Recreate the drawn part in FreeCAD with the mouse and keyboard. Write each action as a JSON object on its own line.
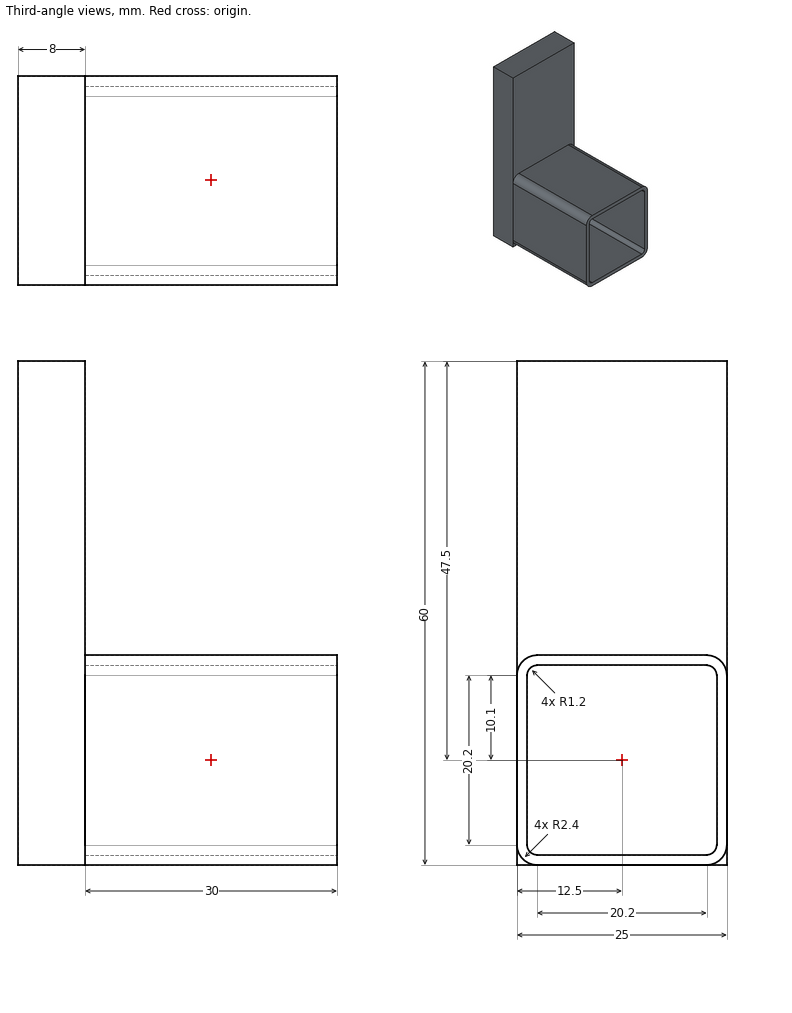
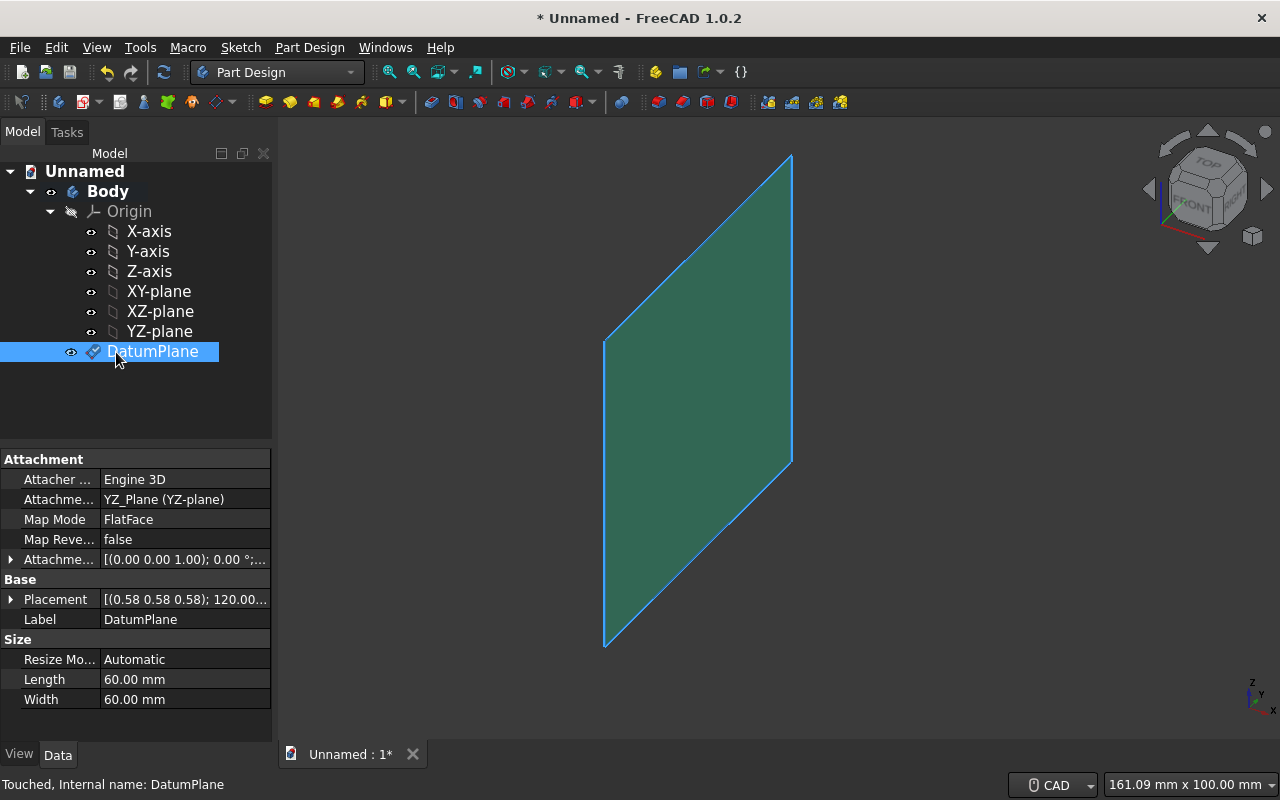
{"action": "left_click", "coordinate": [84, 102]}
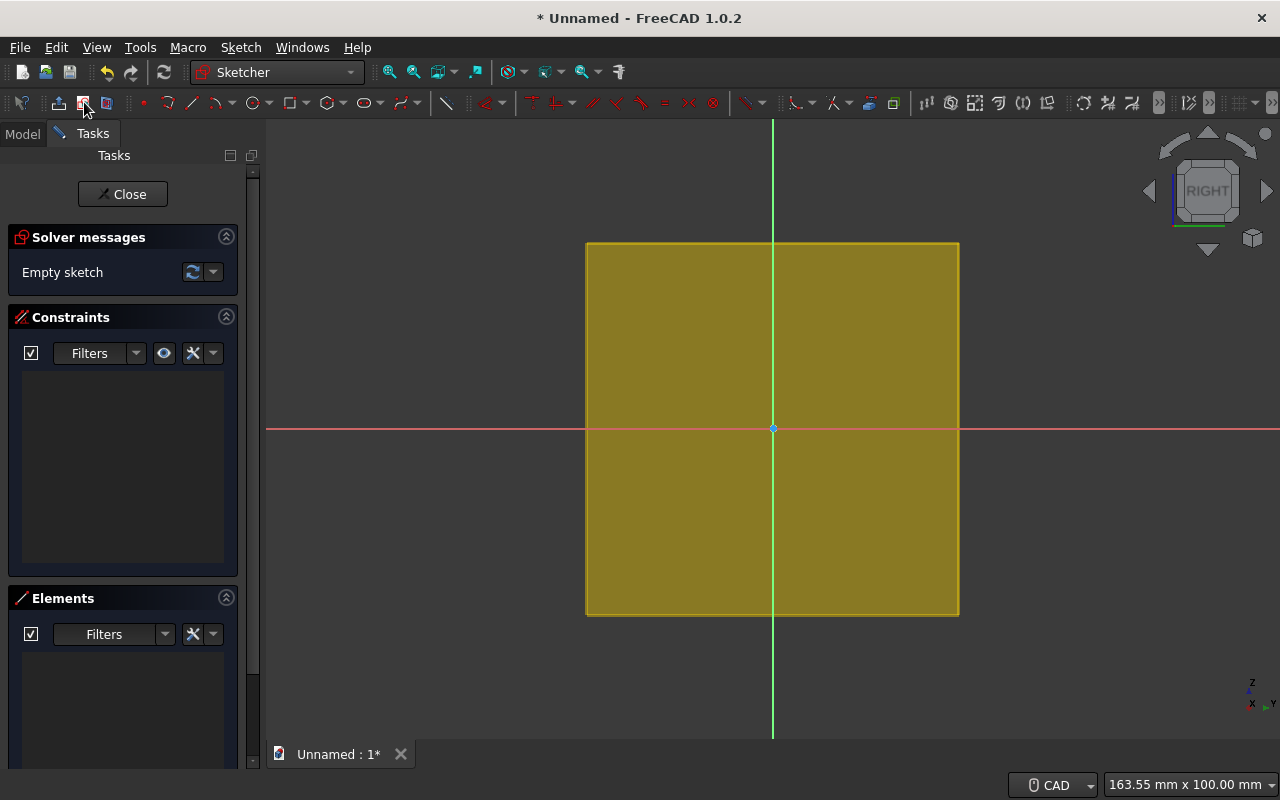
{"action": "scroll", "coordinate": [813, 429], "scroll_direction": "up", "scroll_amount": 5}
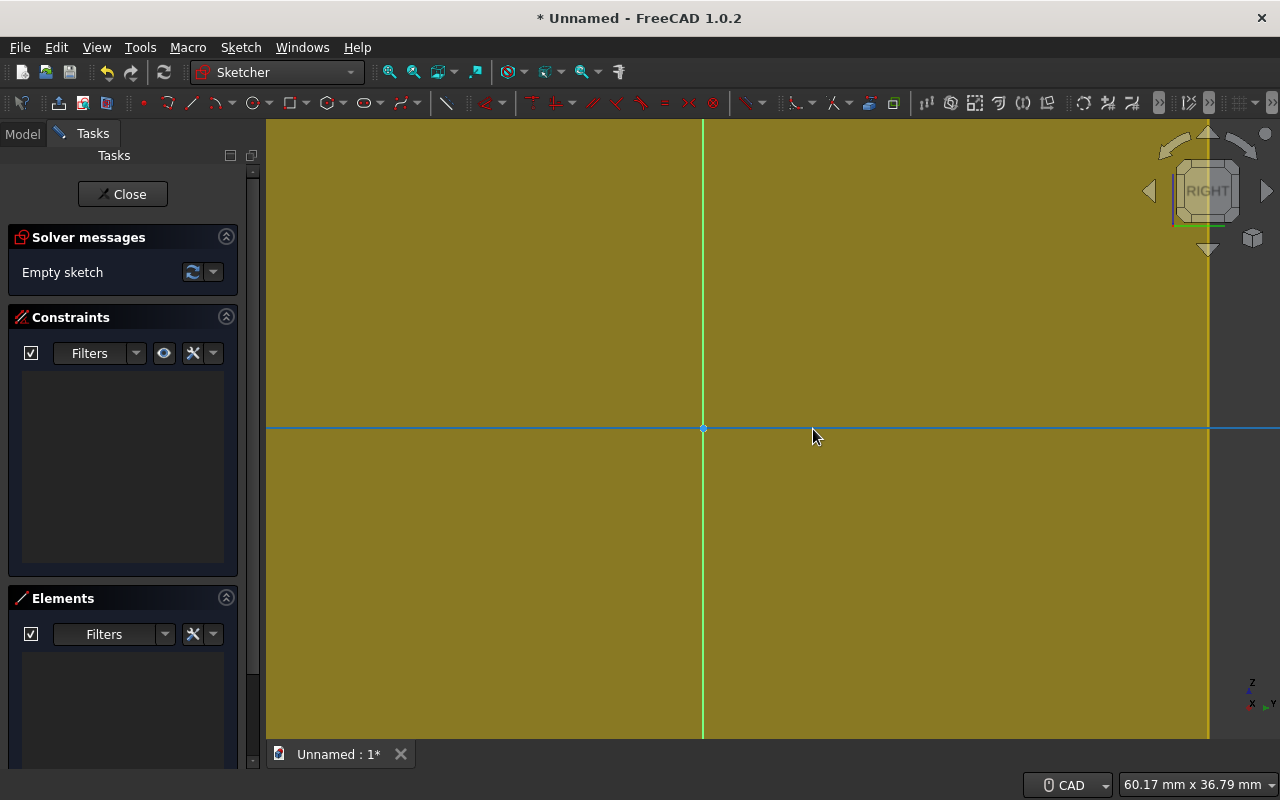
{"action": "left_click", "coordinate": [192, 104]}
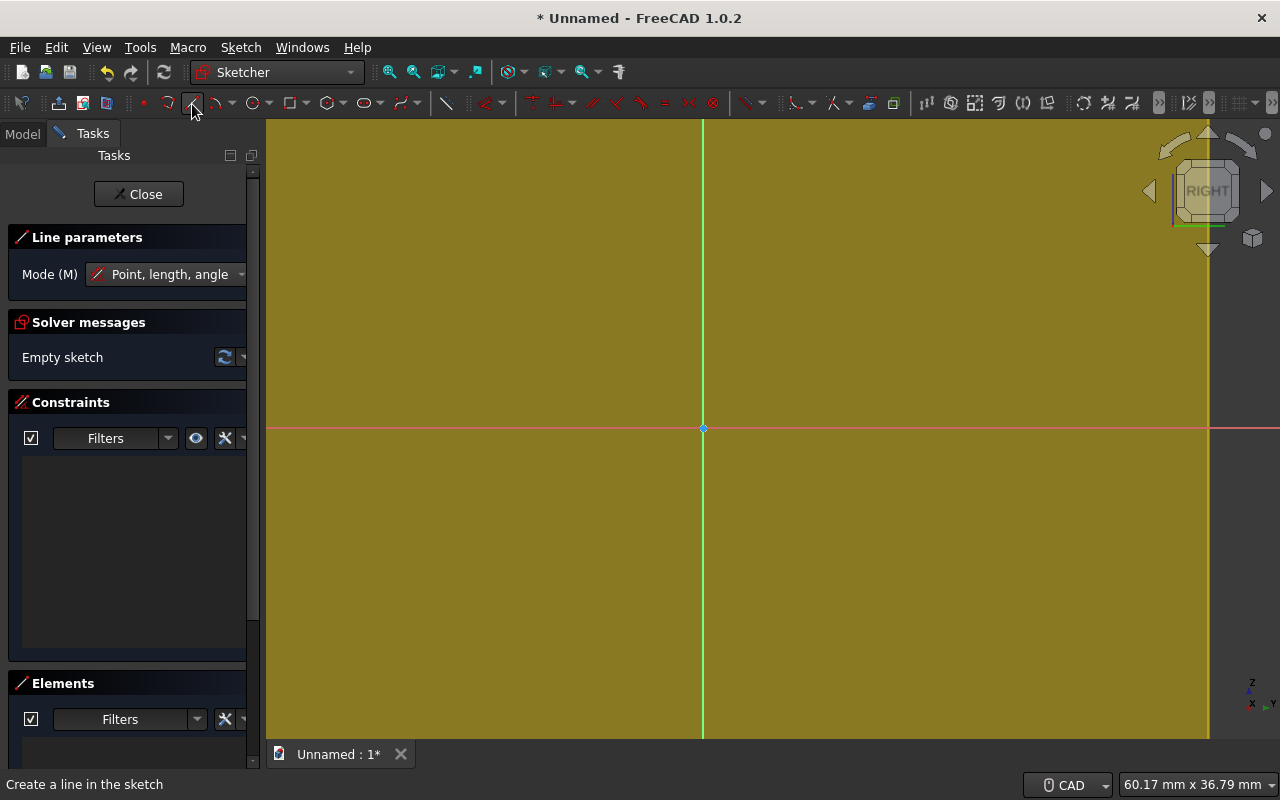
{"action": "left_click", "coordinate": [493, 258]}
{"action": "left_click", "coordinate": [493, 598]}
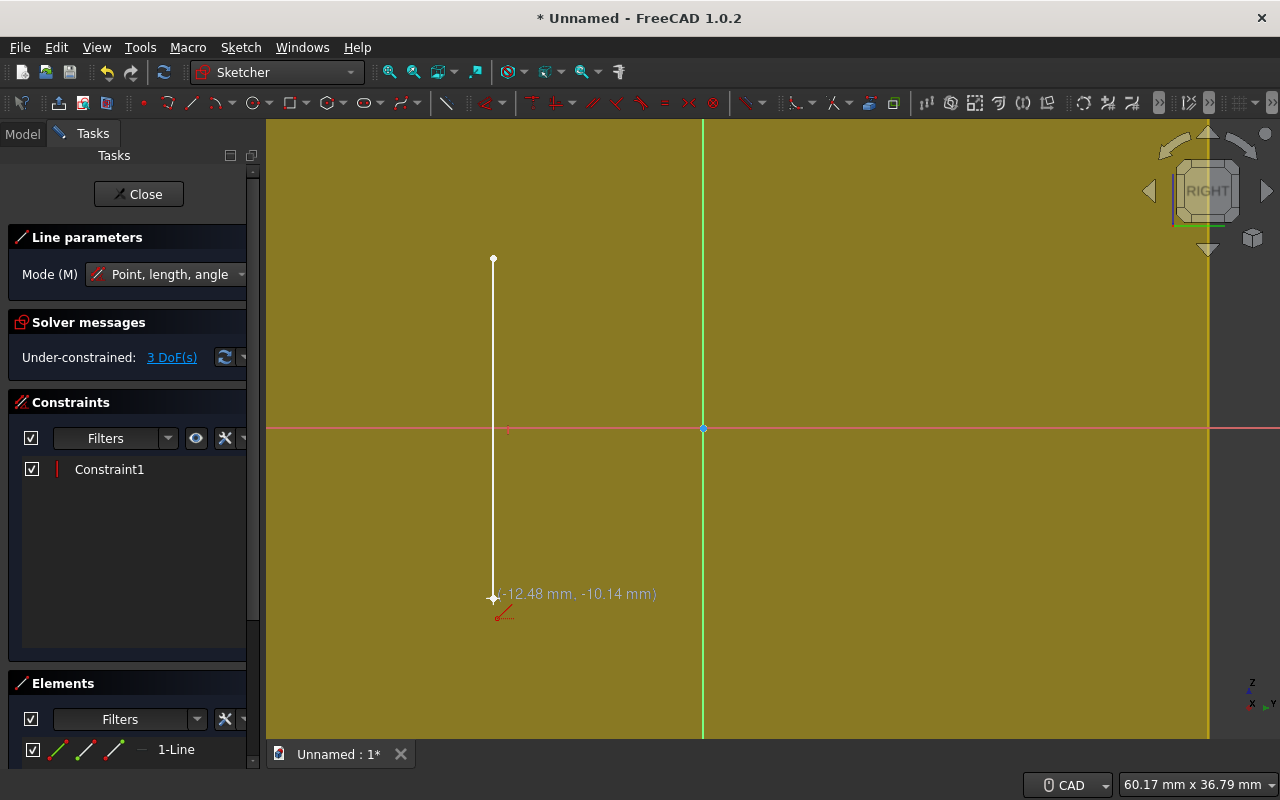
{"action": "left_click", "coordinate": [533, 639]}
{"action": "left_click", "coordinate": [874, 639]}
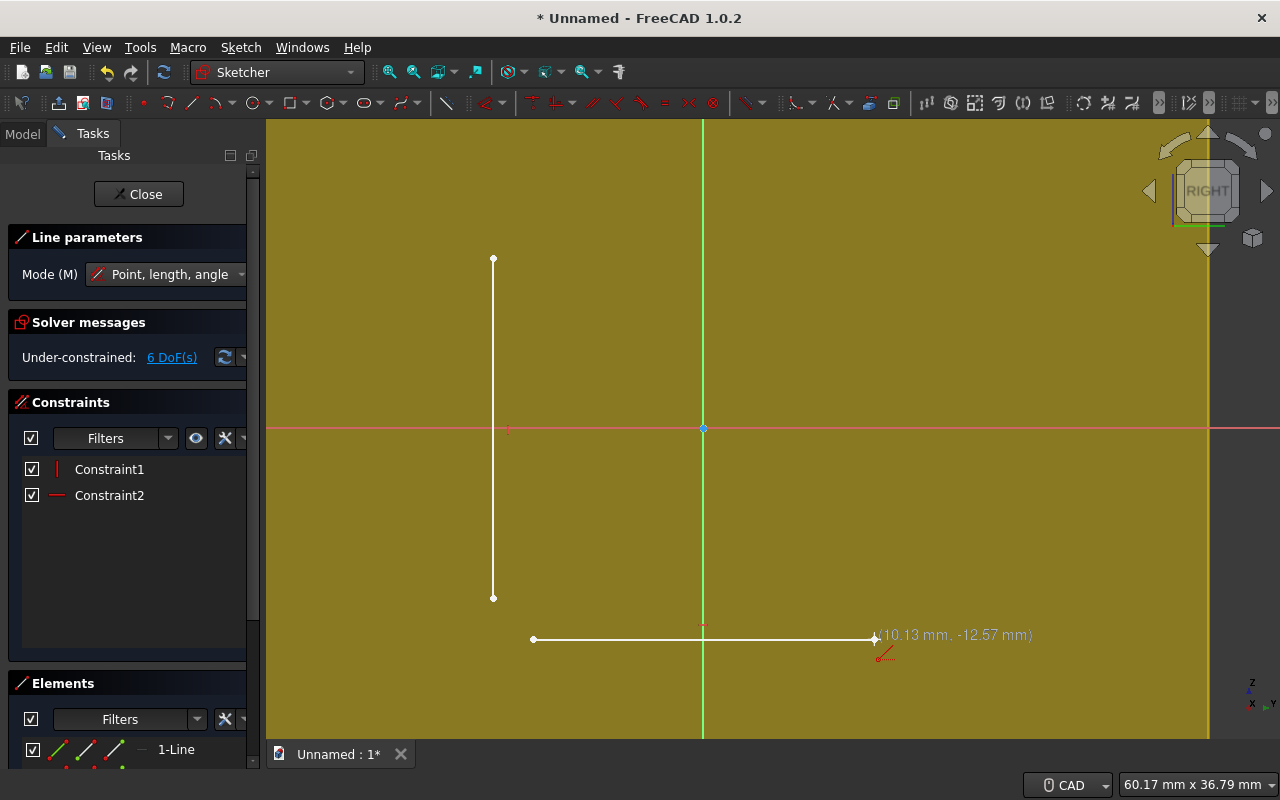
{"action": "left_click", "coordinate": [914, 598]}
{"action": "left_click", "coordinate": [914, 258]}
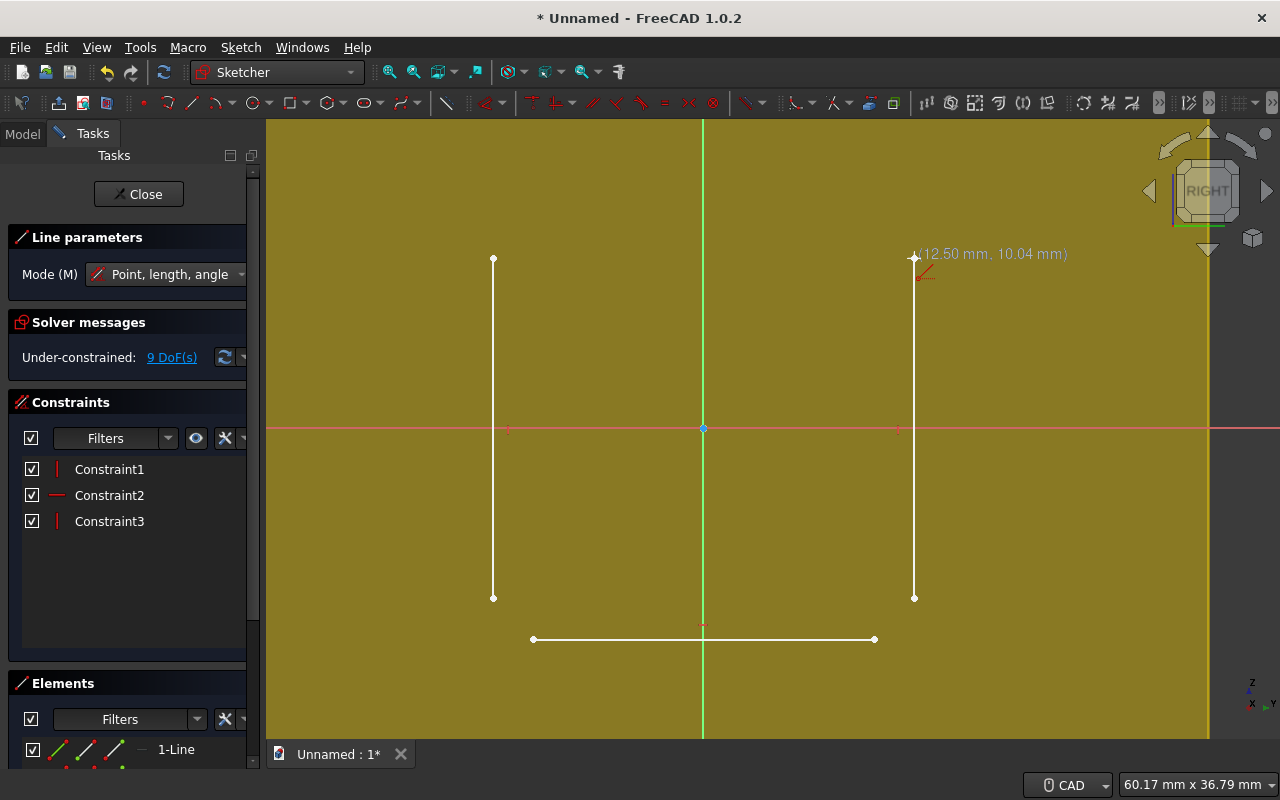
{"action": "left_click", "coordinate": [874, 217]}
{"action": "left_click", "coordinate": [533, 217]}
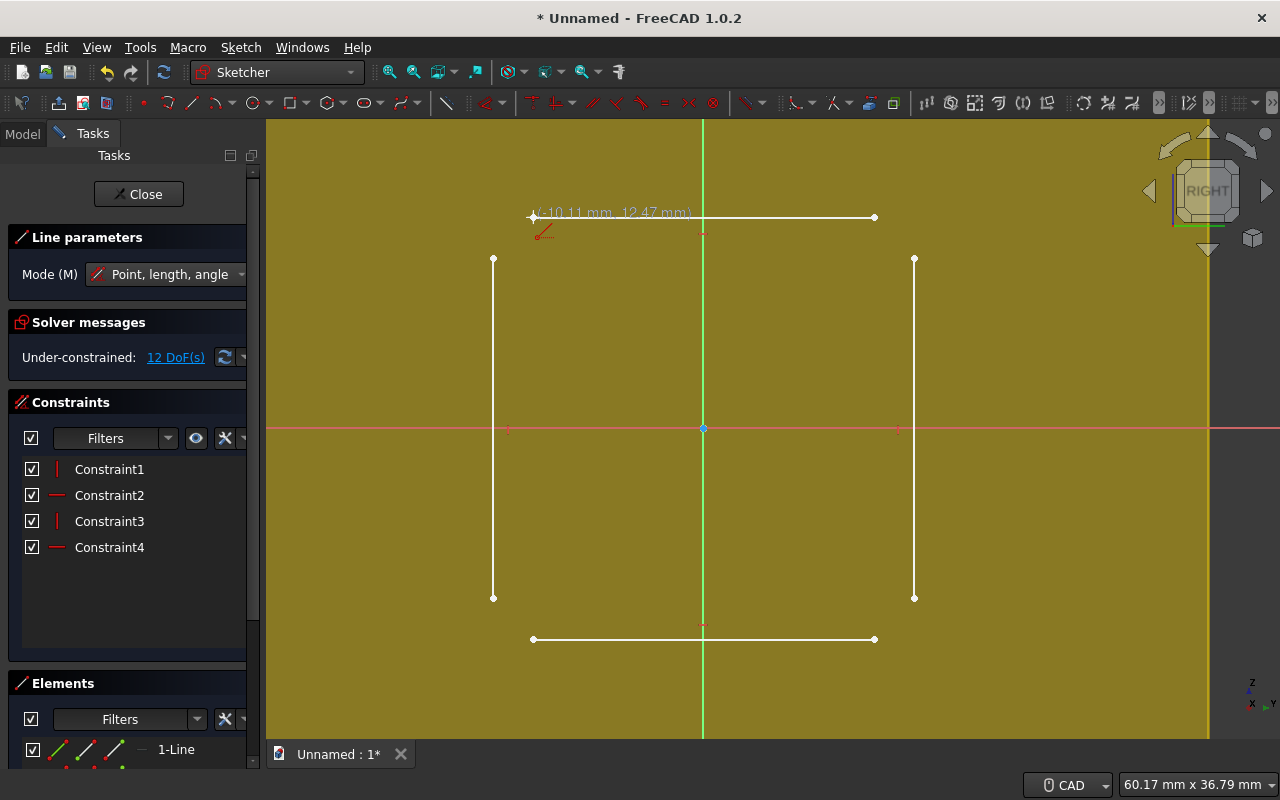
{"action": "left_click", "coordinate": [234, 104]}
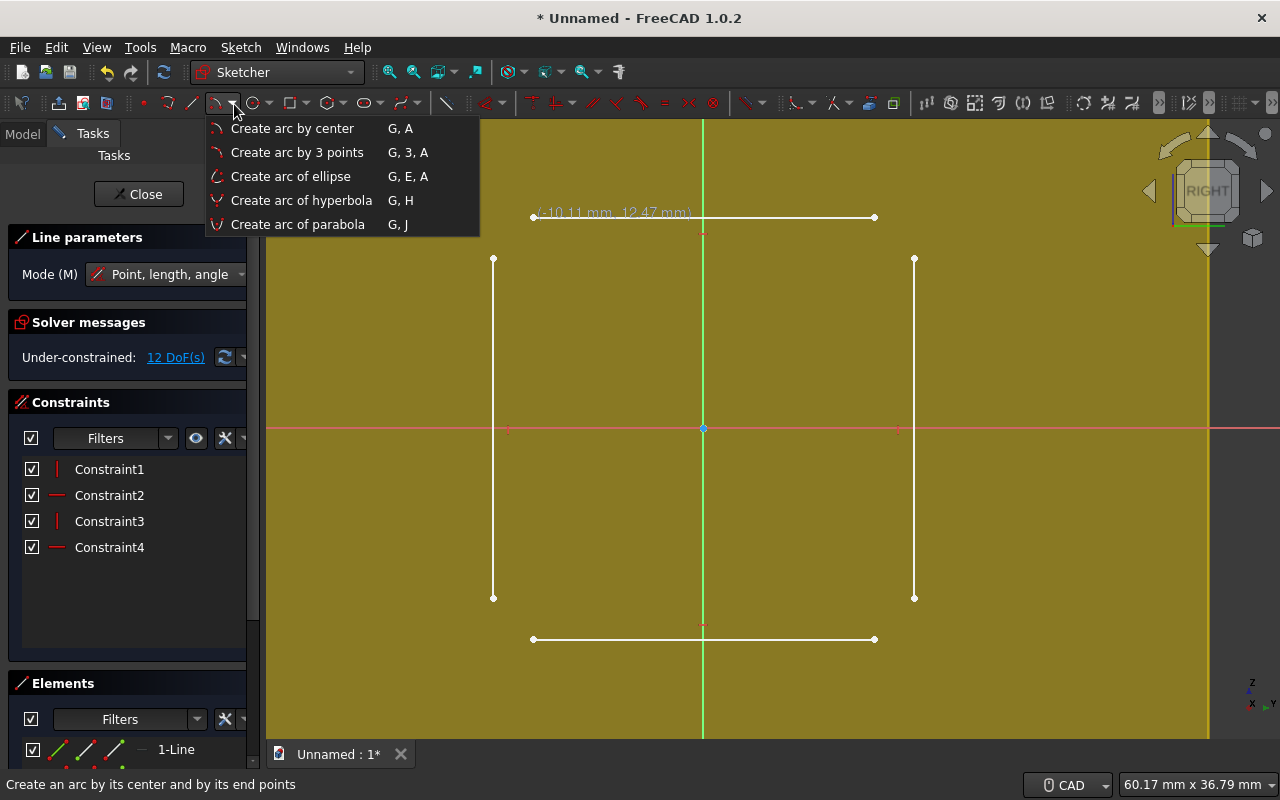
{"action": "left_click", "coordinate": [342, 152]}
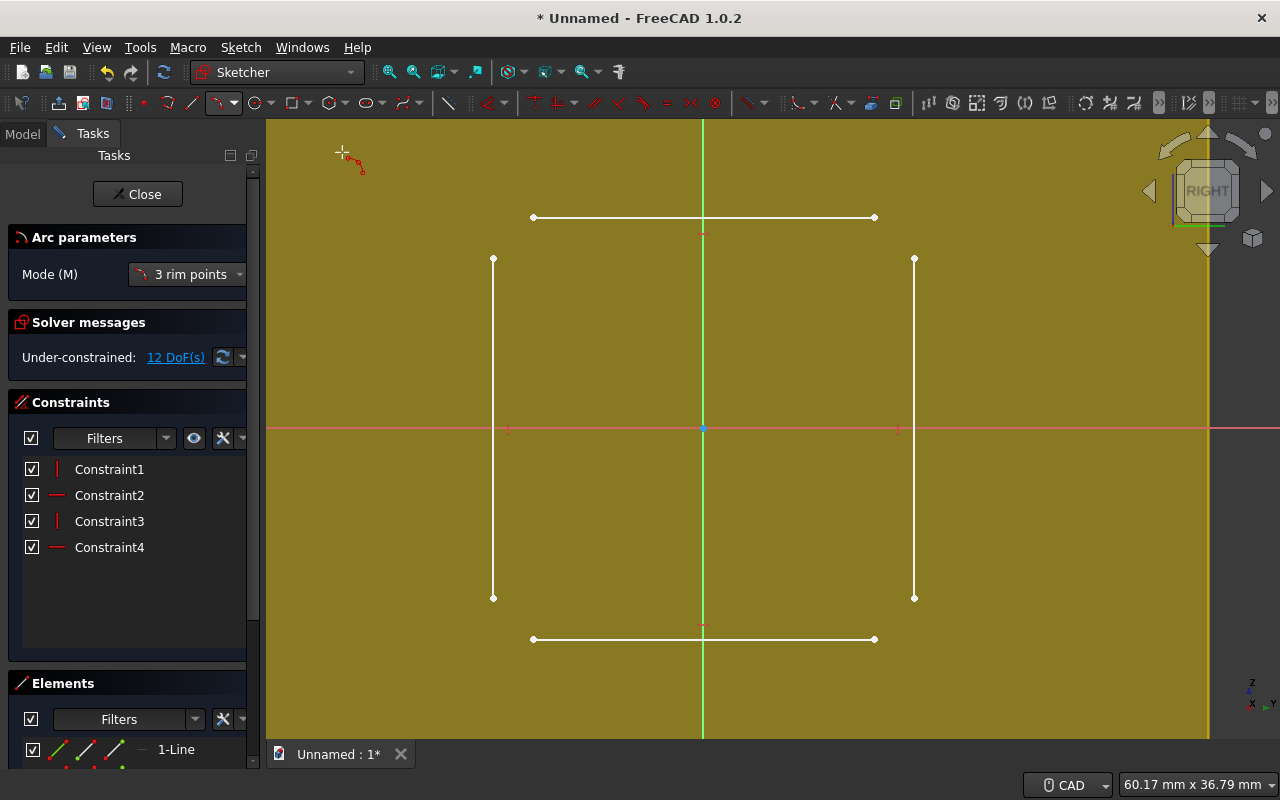
{"action": "left_click", "coordinate": [493, 599]}
{"action": "left_click", "coordinate": [533, 640]}